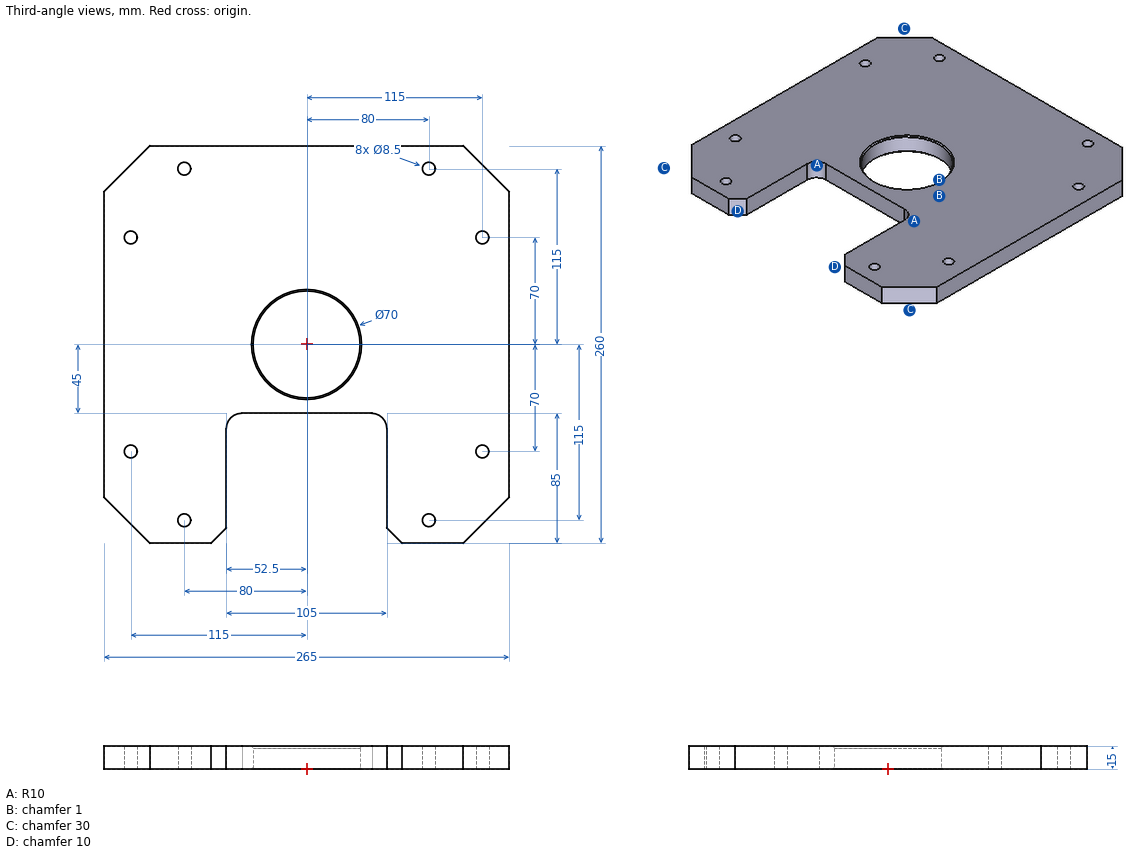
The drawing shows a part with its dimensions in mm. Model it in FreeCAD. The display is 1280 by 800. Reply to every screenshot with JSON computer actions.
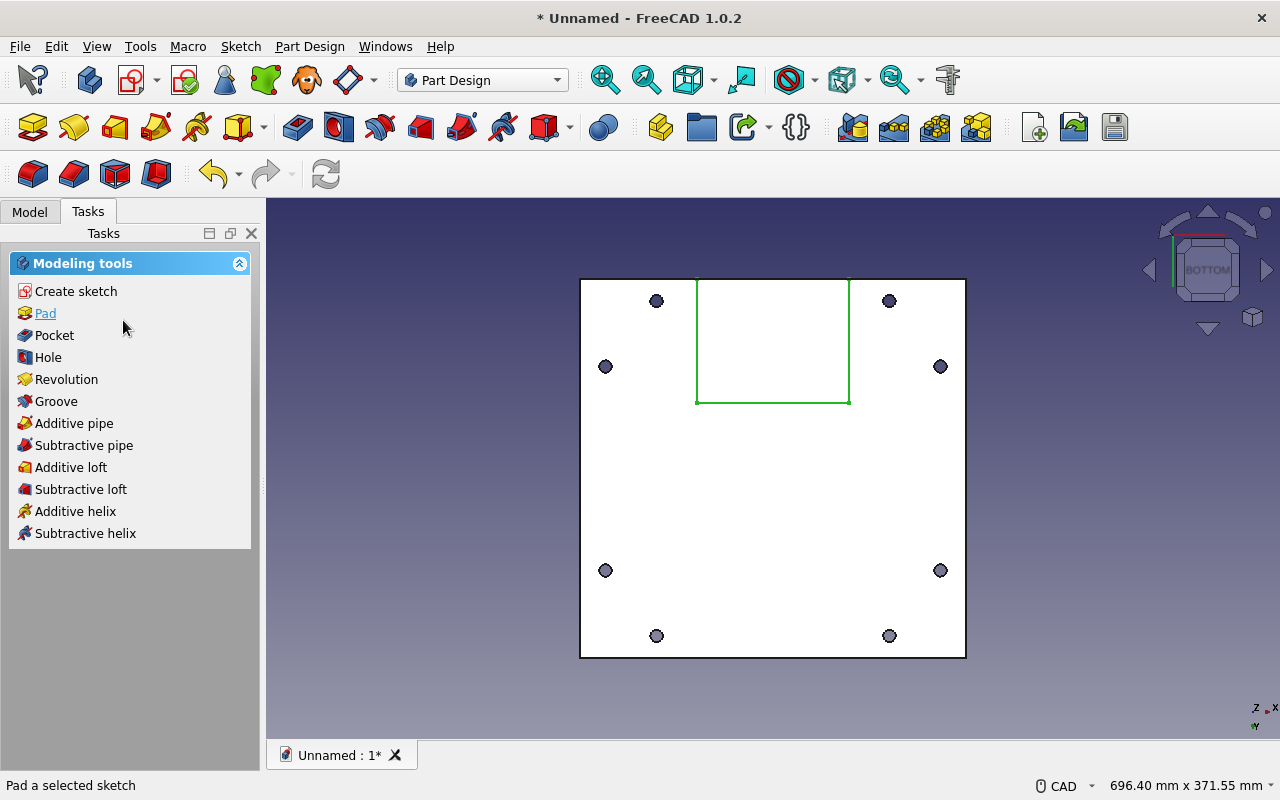
{"action": "left_click", "coordinate": [298, 128]}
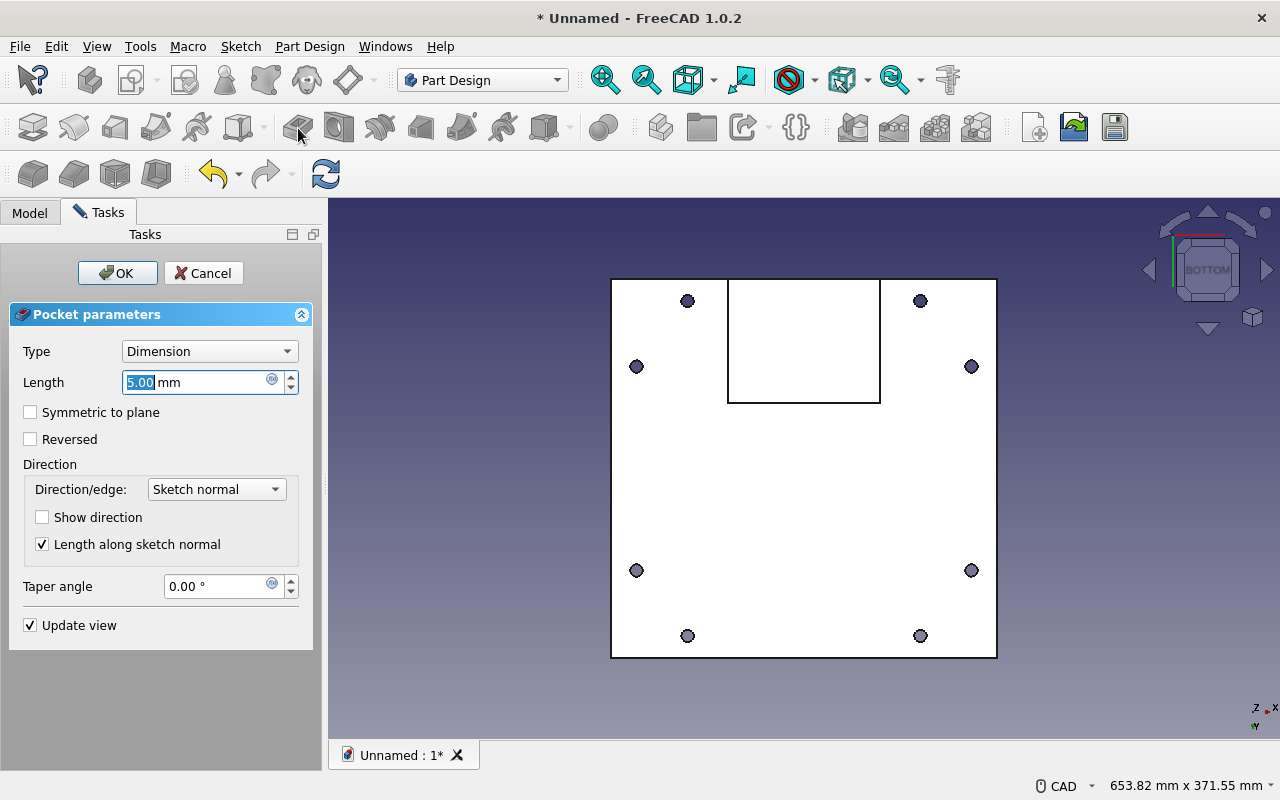
{"action": "left_click", "coordinate": [210, 352]}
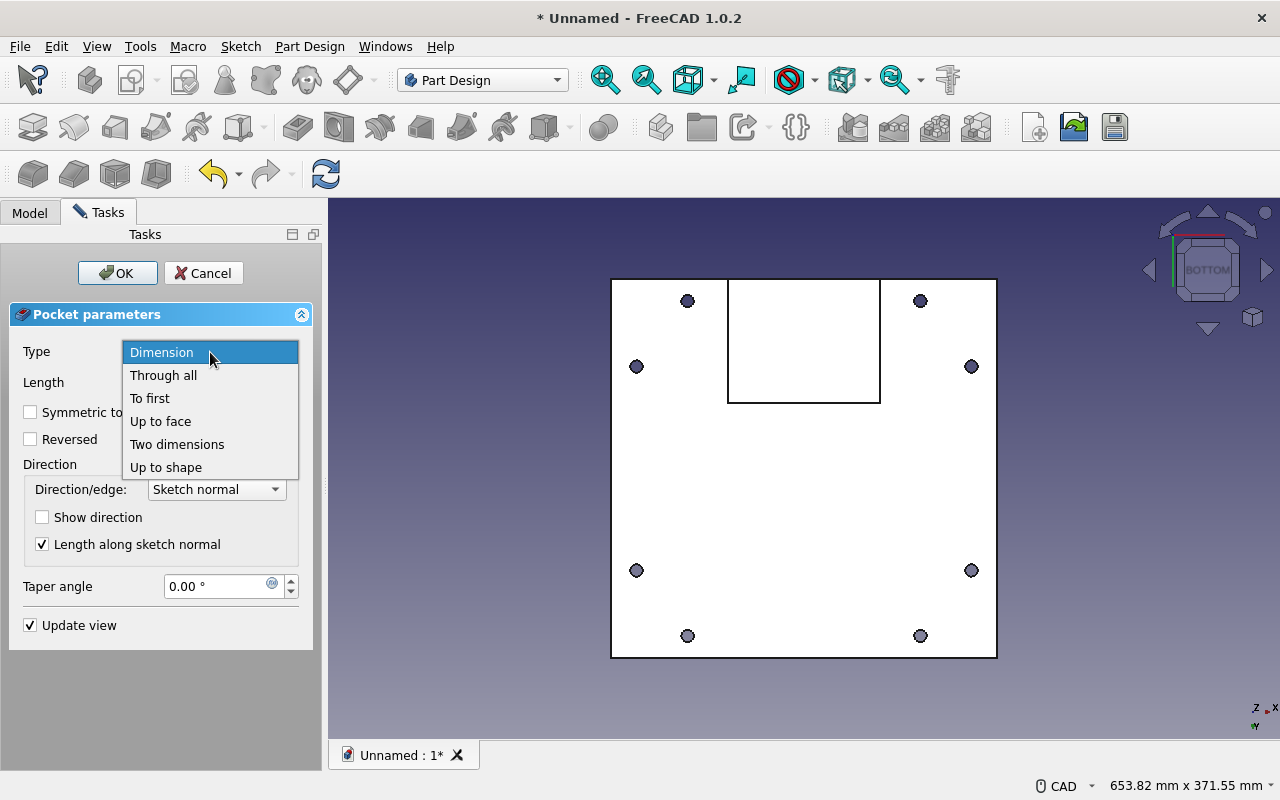
{"action": "left_click", "coordinate": [208, 376]}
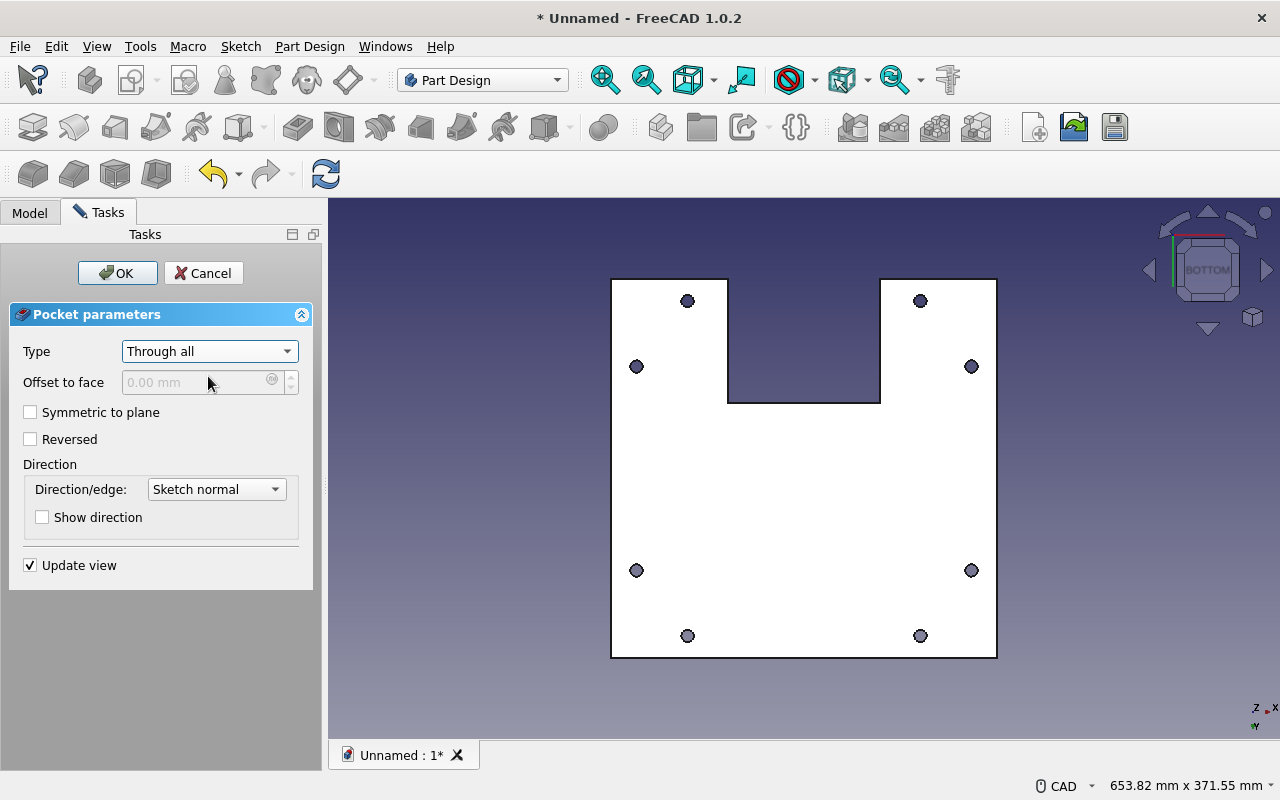
{"action": "left_click", "coordinate": [118, 273]}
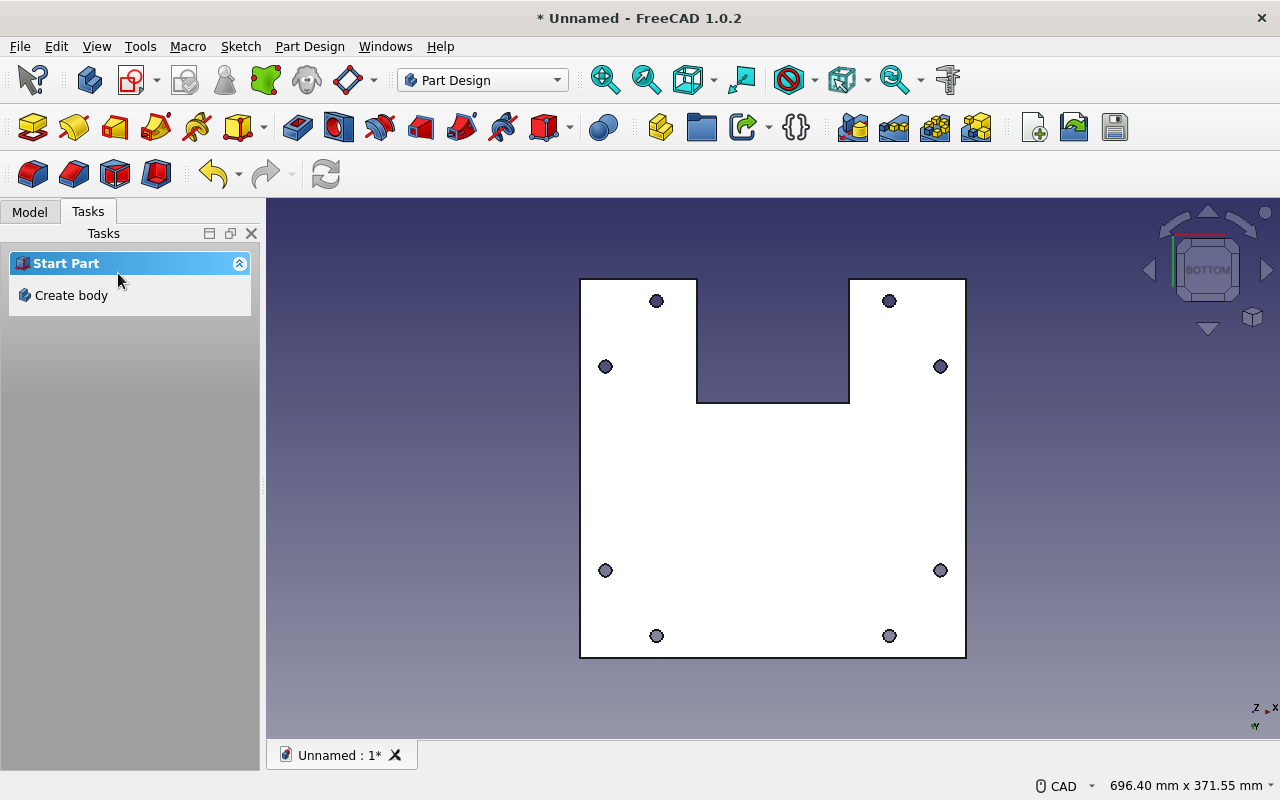
{"action": "scroll", "coordinate": [849, 402], "scroll_direction": "up", "scroll_amount": 4}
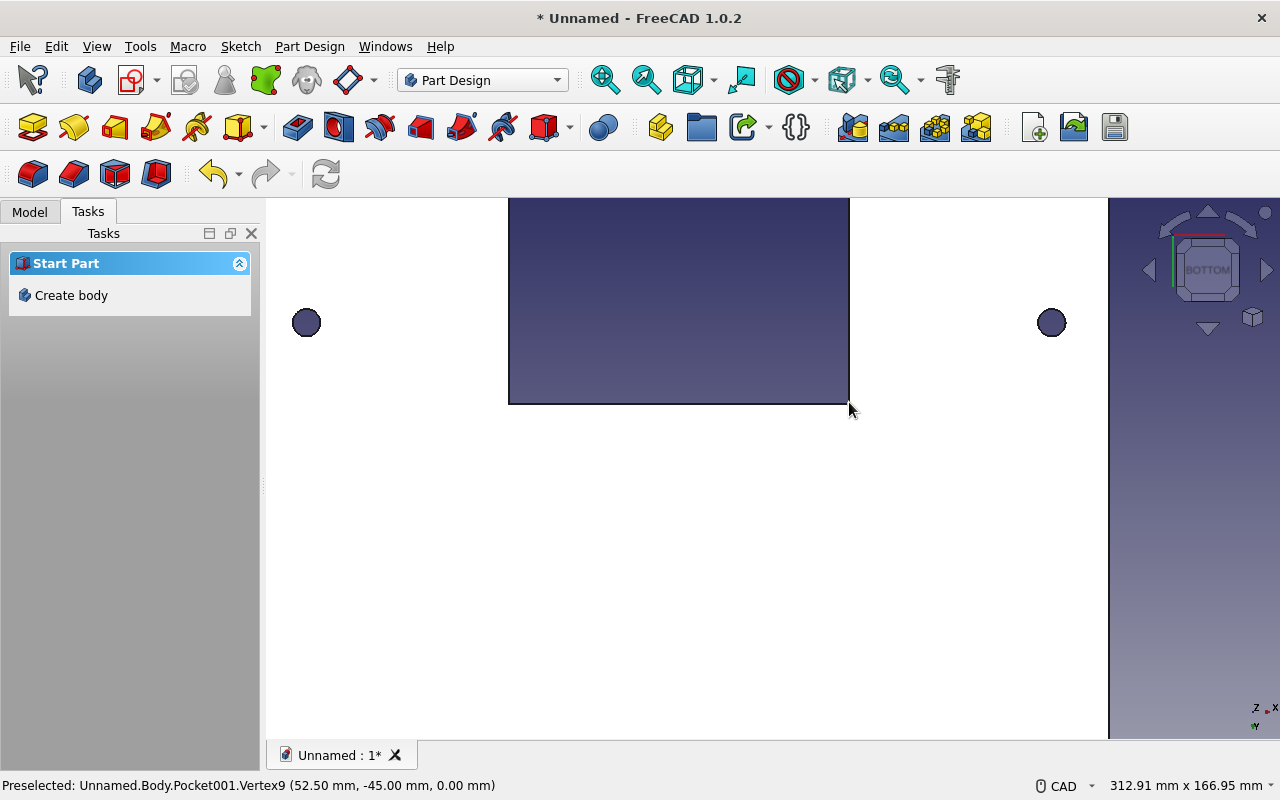
{"action": "left_click", "coordinate": [606, 80]}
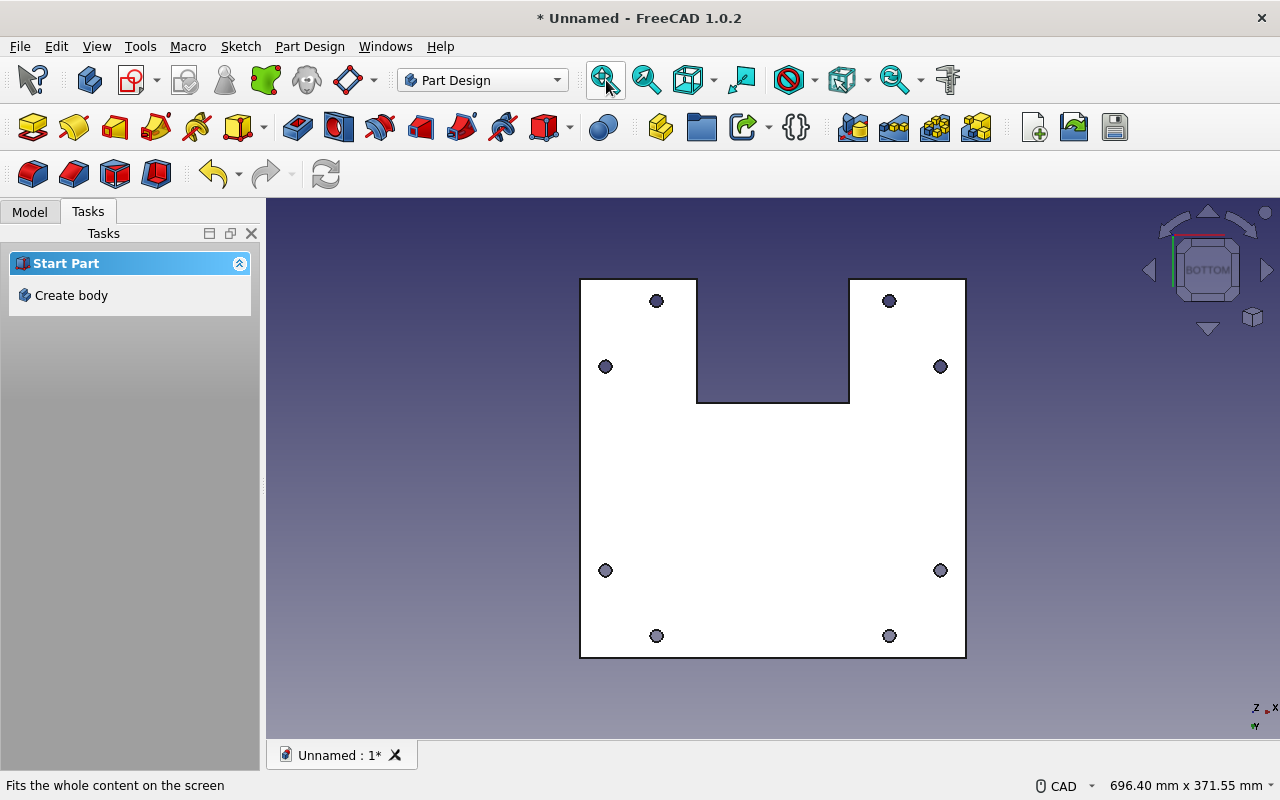
{"action": "key", "text": "0"}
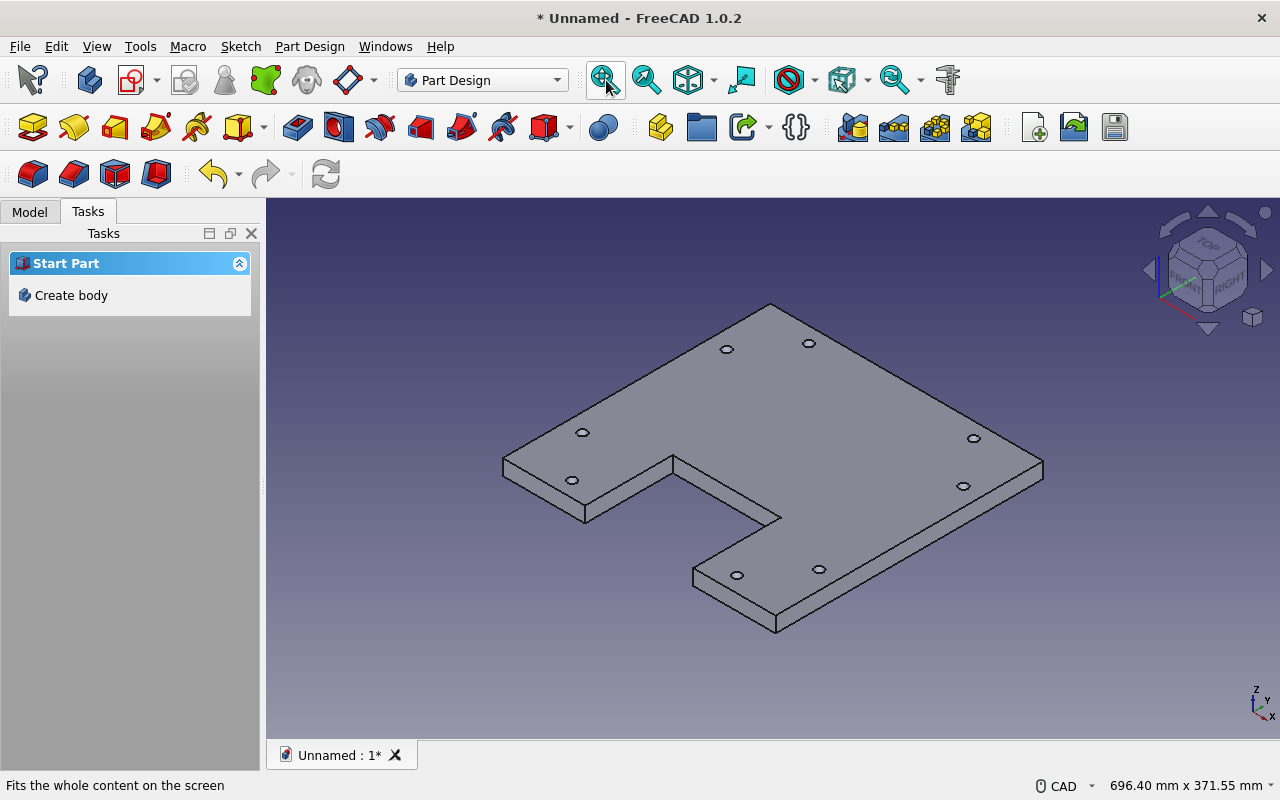
{"action": "scroll", "coordinate": [781, 525], "scroll_direction": "up", "scroll_amount": 4}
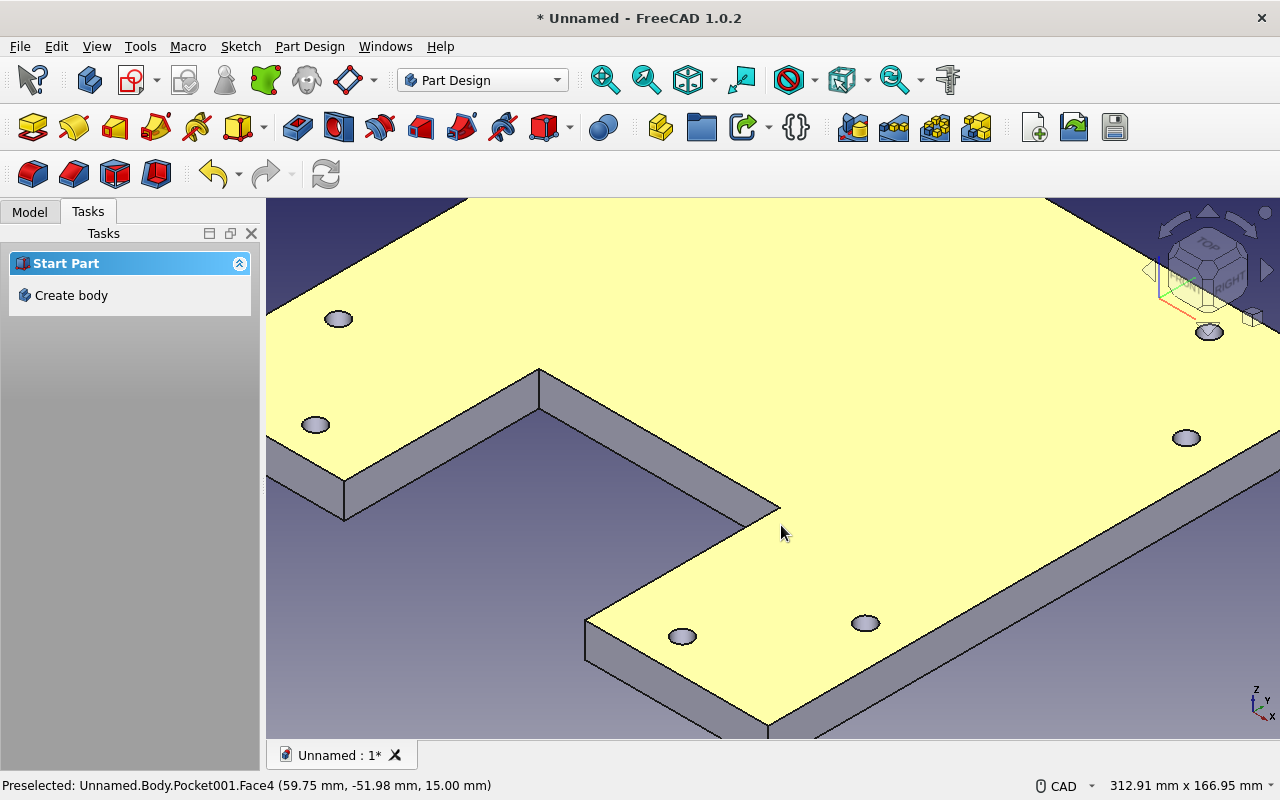
{"action": "left_click", "coordinate": [606, 80]}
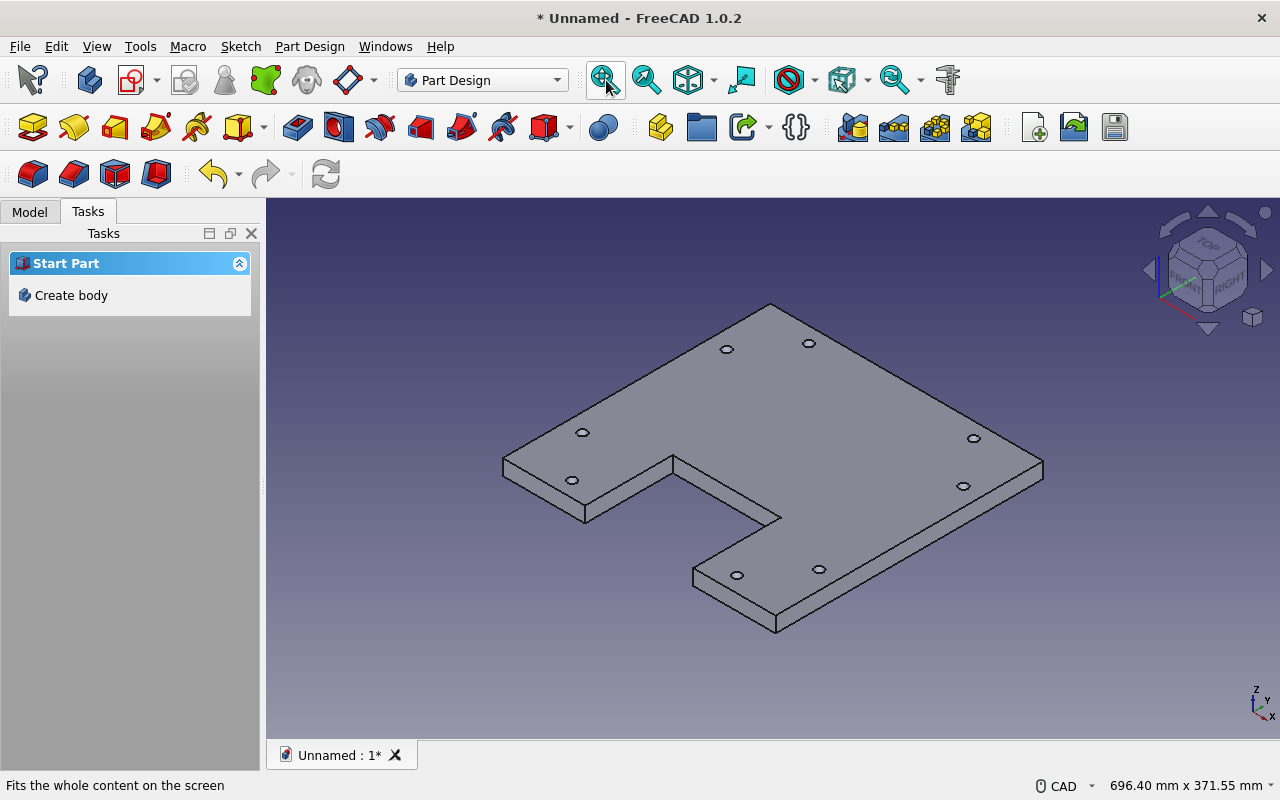
{"action": "key", "text": "2"}